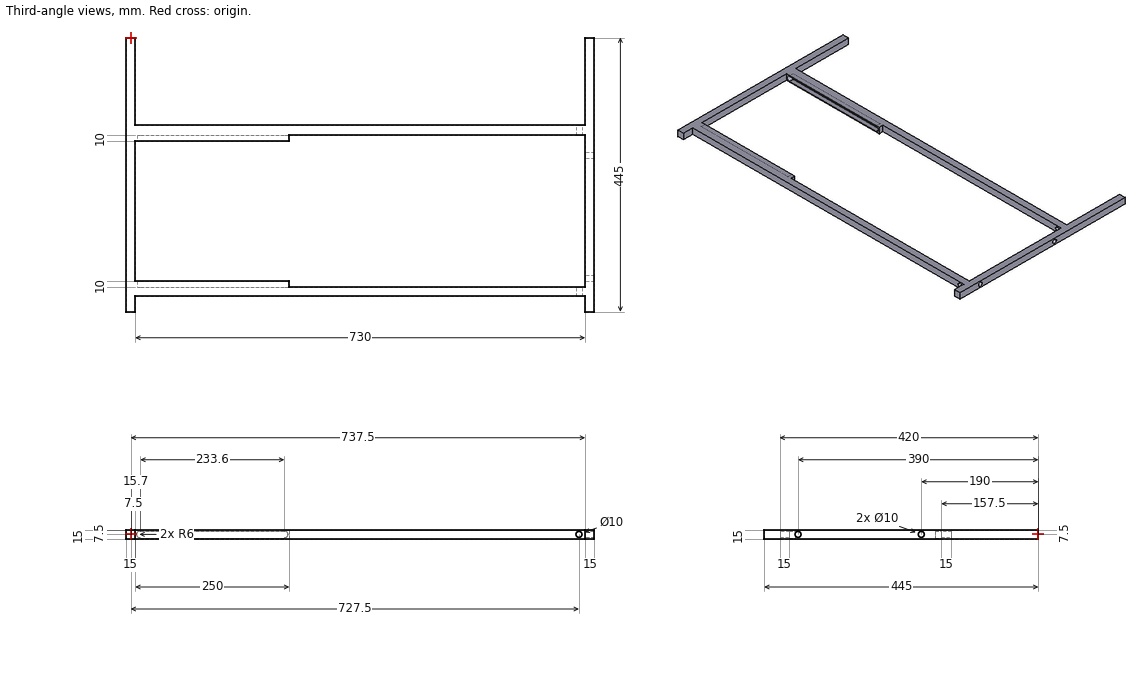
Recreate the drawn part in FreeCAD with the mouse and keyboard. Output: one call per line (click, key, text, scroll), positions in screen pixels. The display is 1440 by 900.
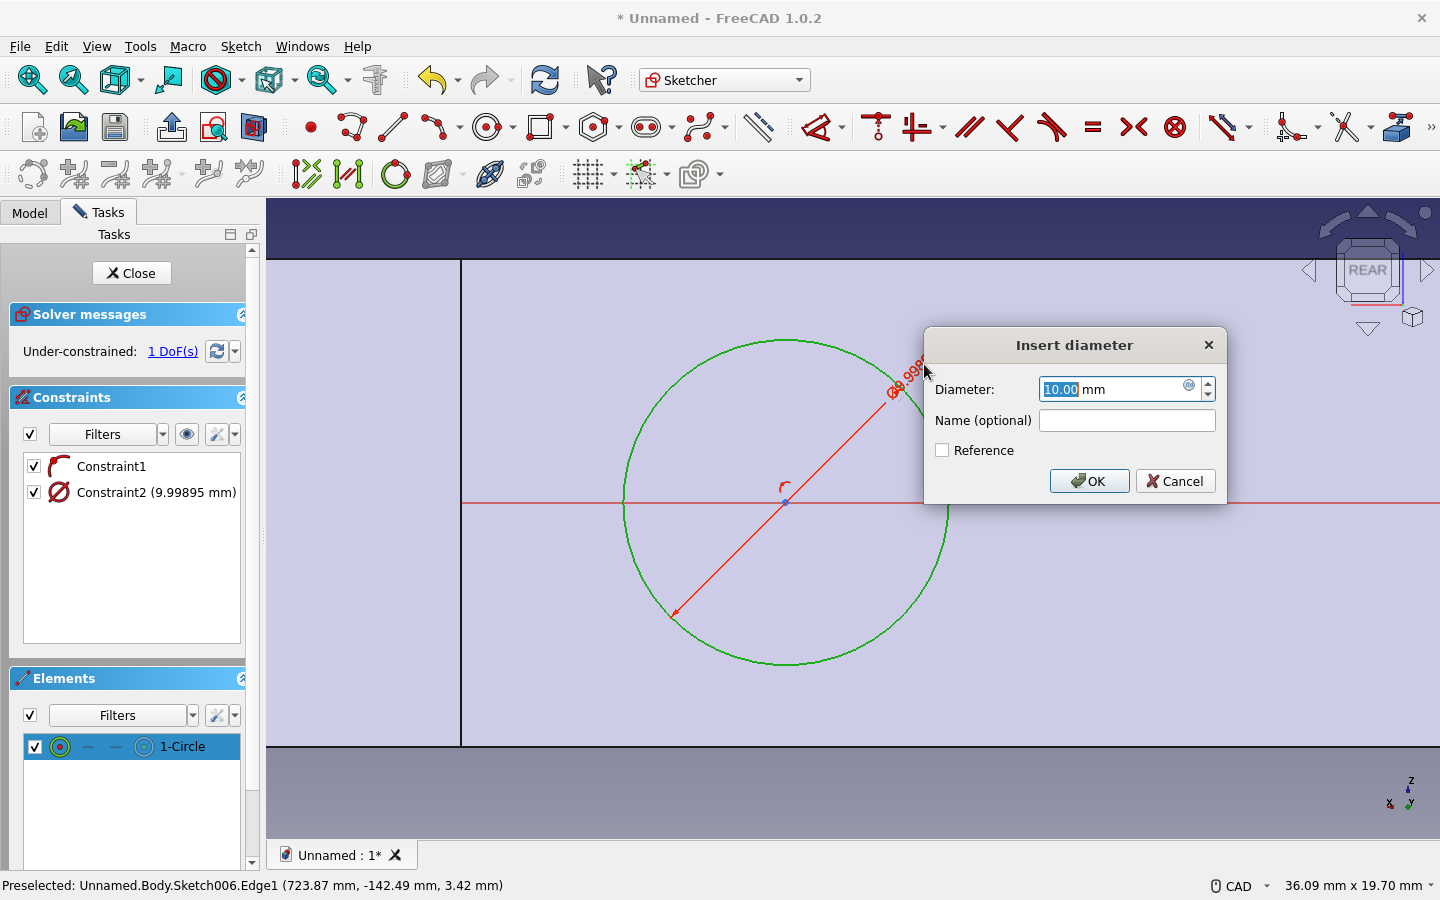
text(10)
key(Return)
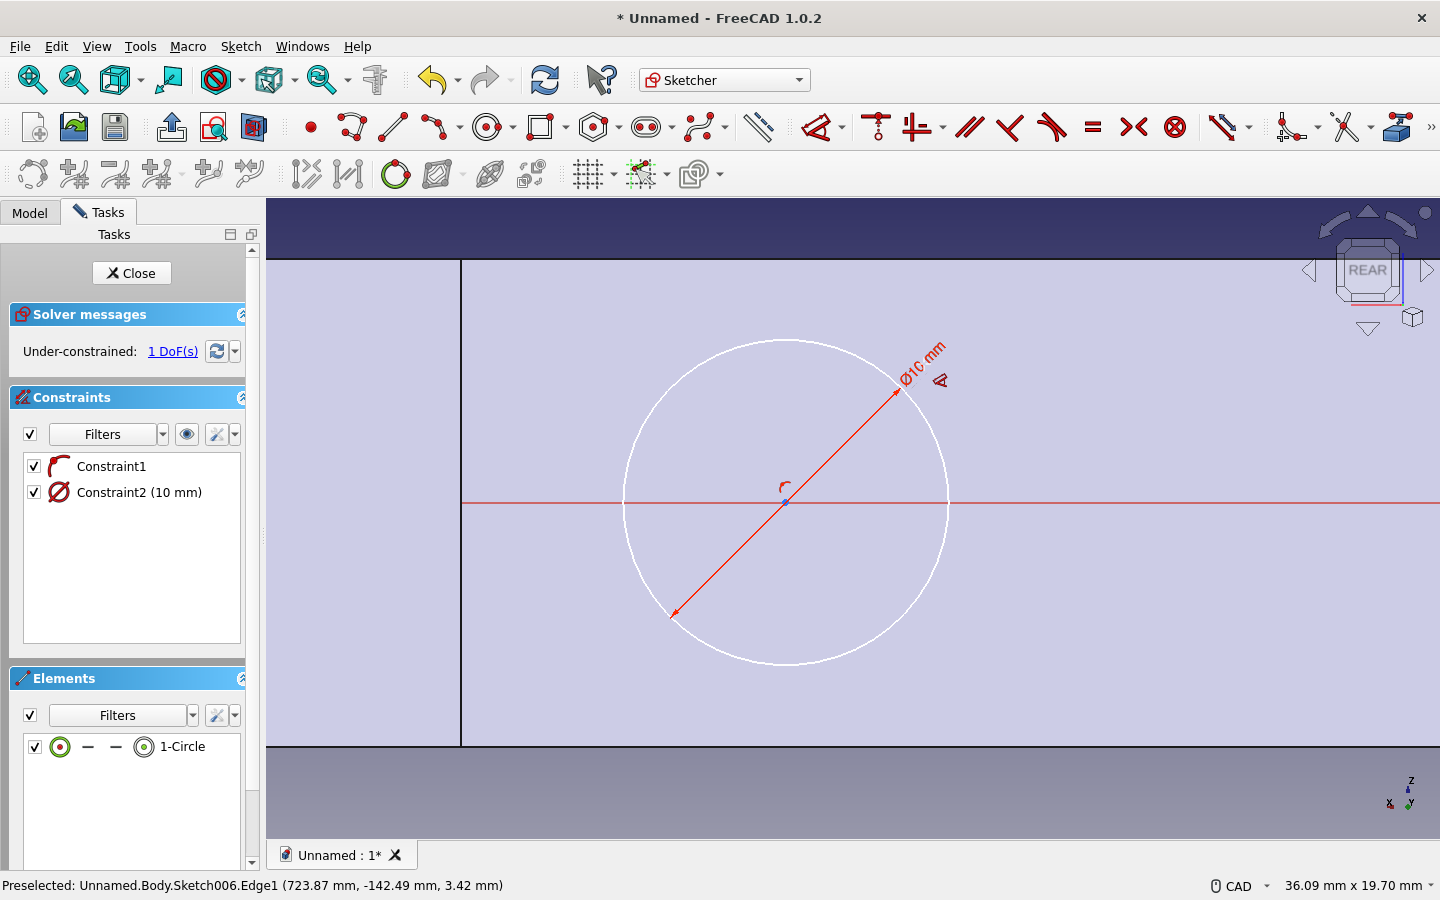
click(786, 503)
click(1030, 537)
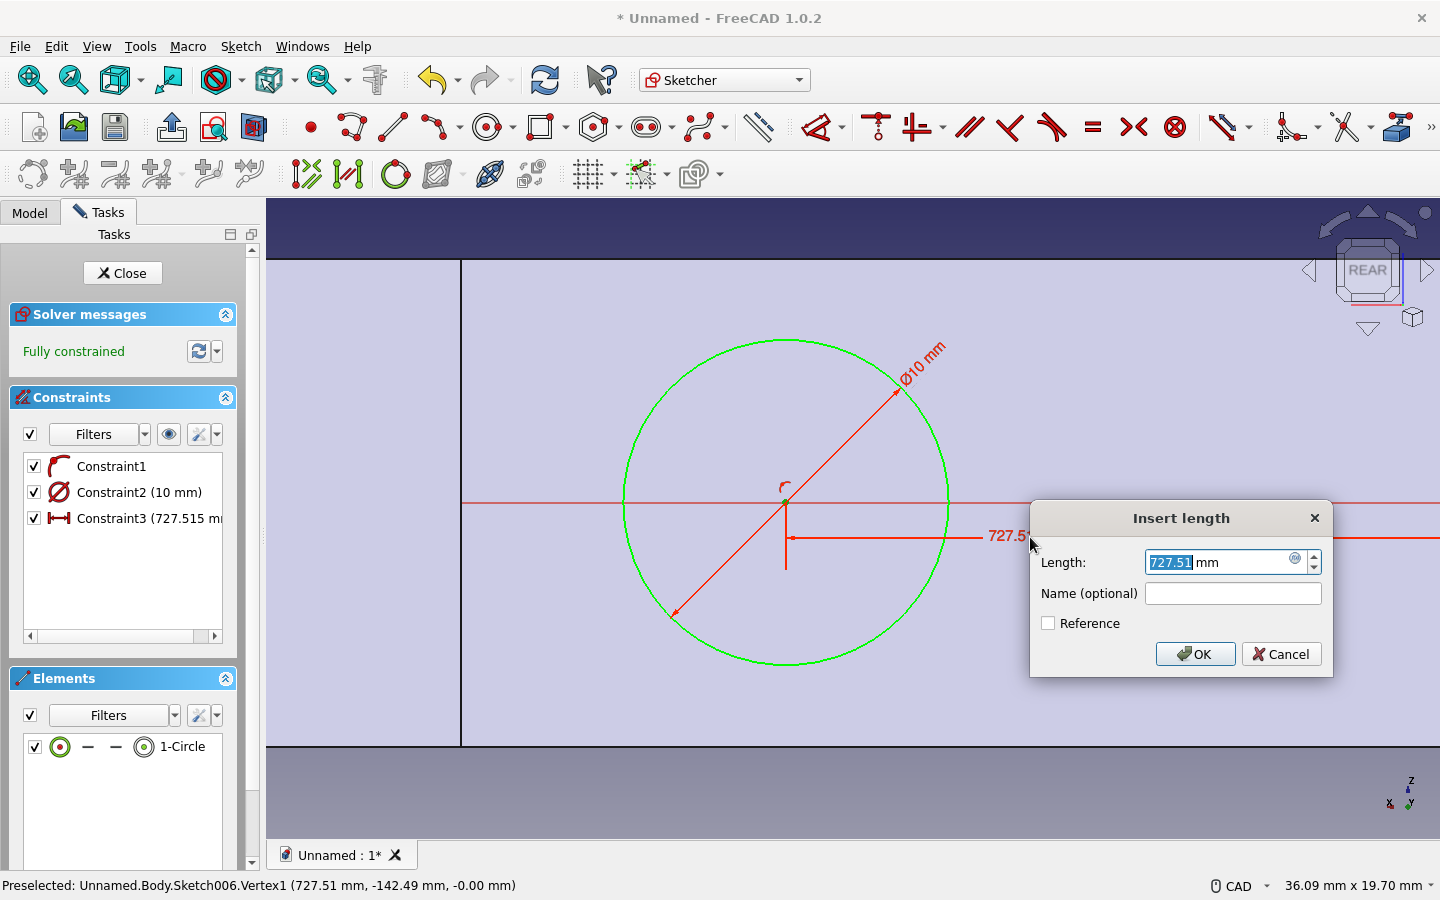
text(727.5)
key(Return)
key(Escape)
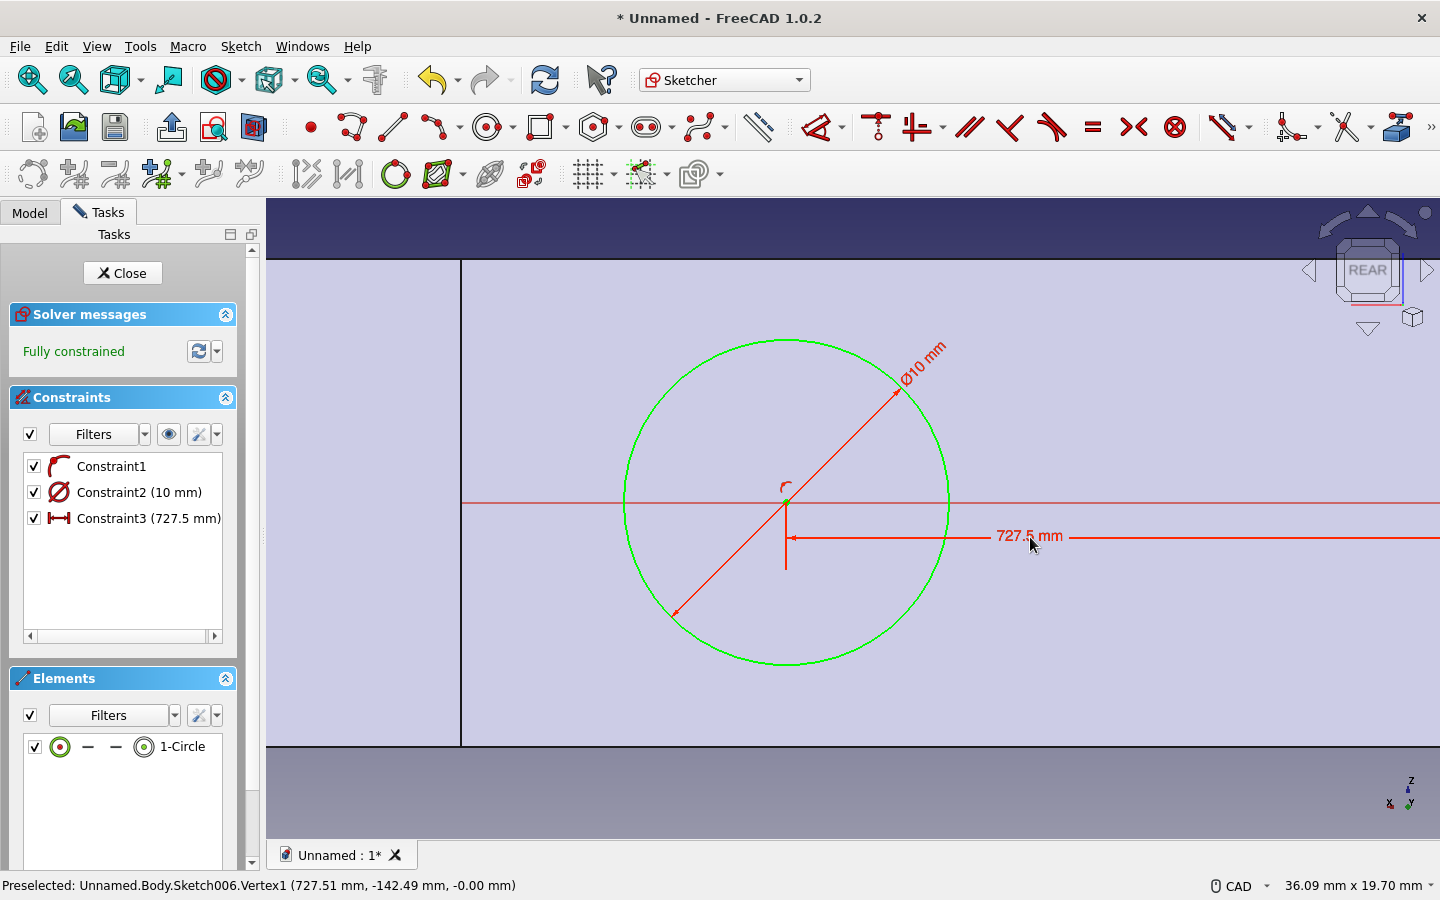
click(123, 273)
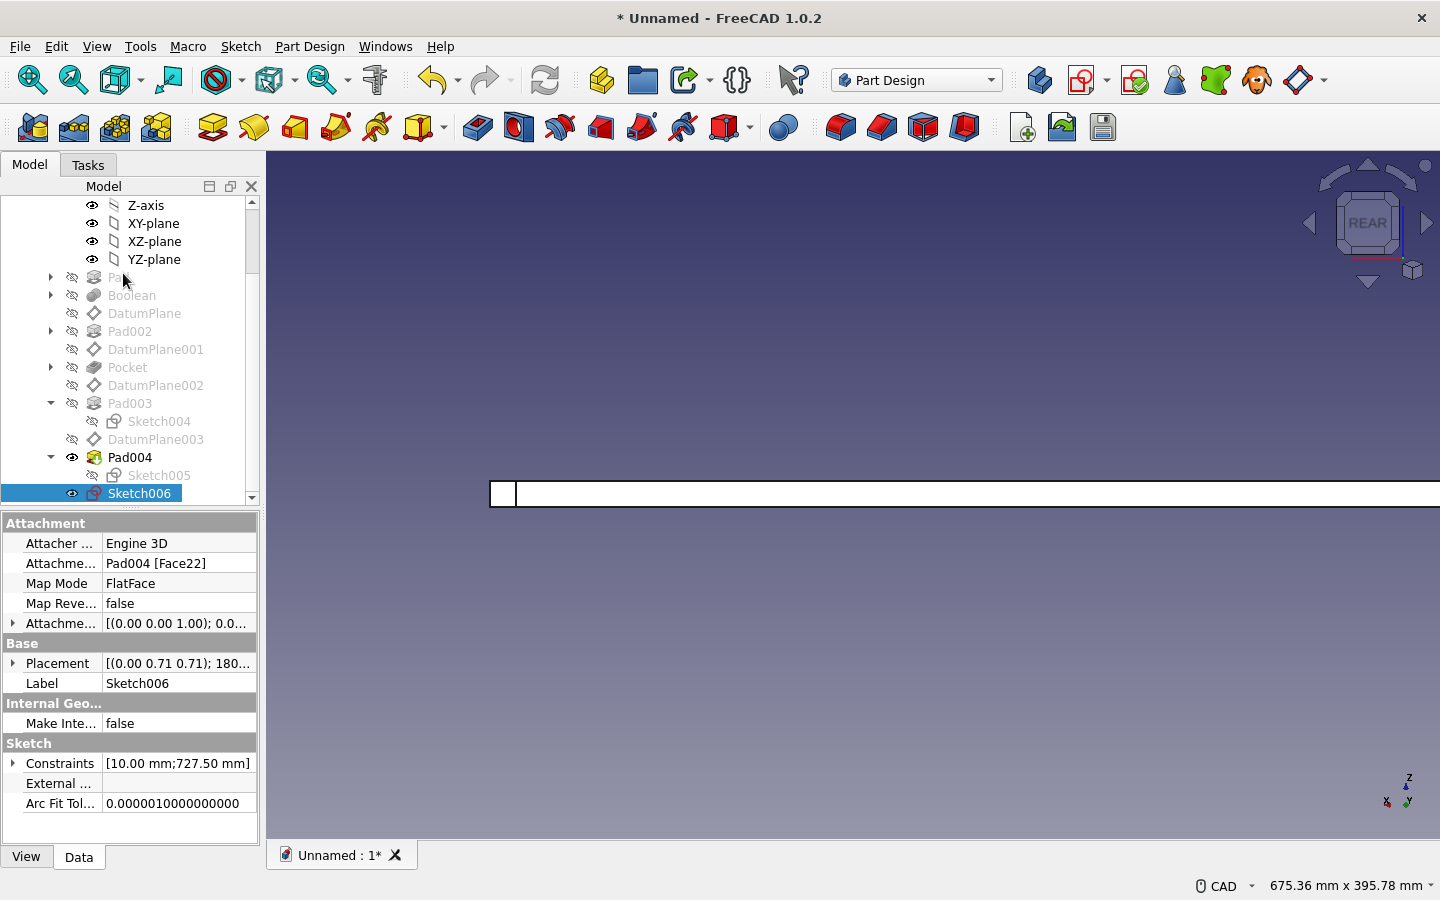
click(478, 128)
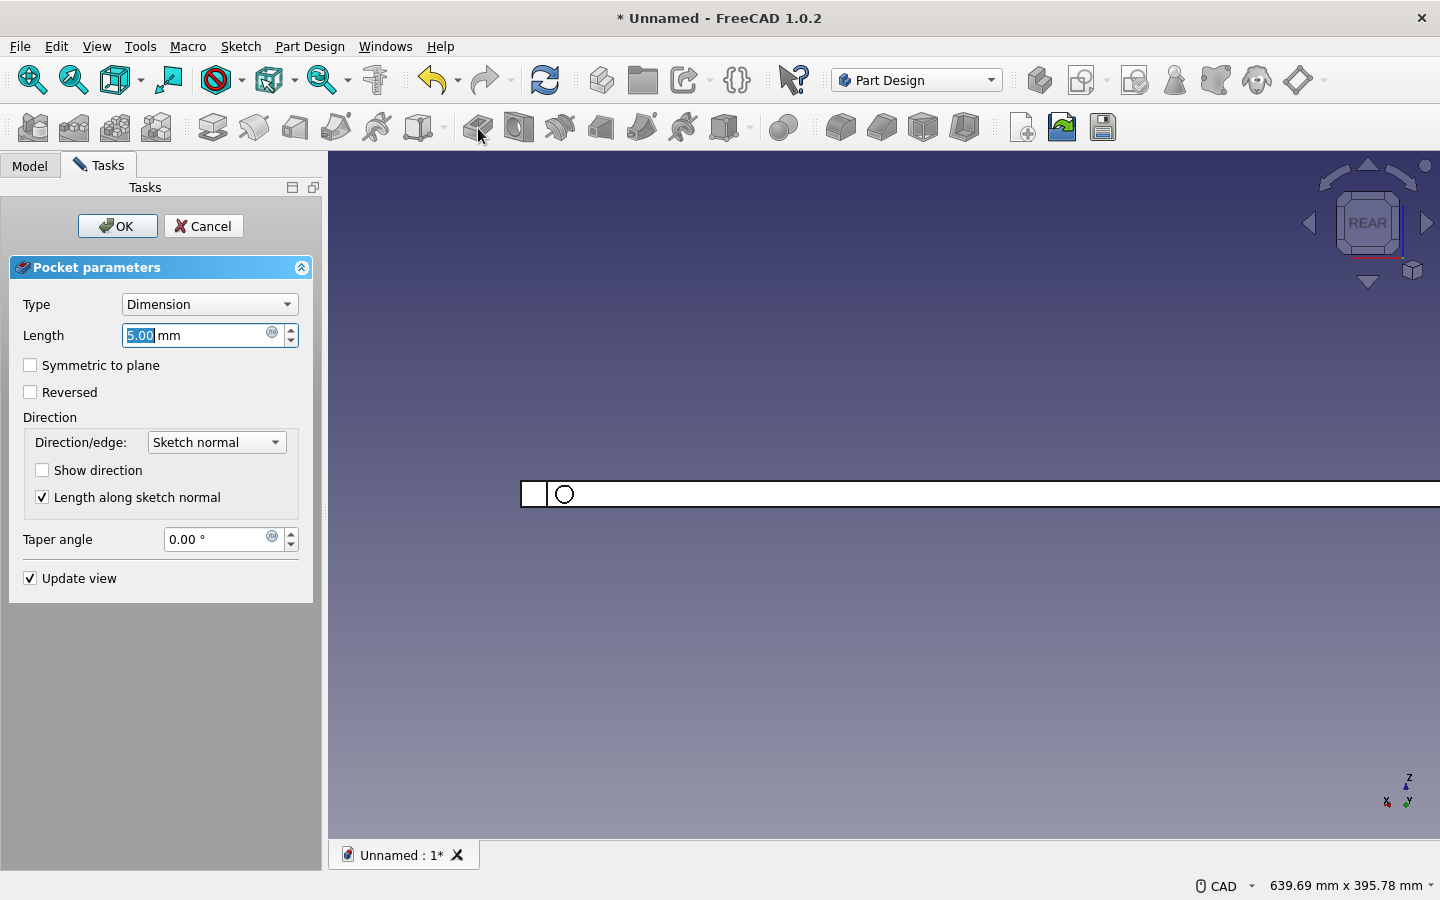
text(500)
key(Tab)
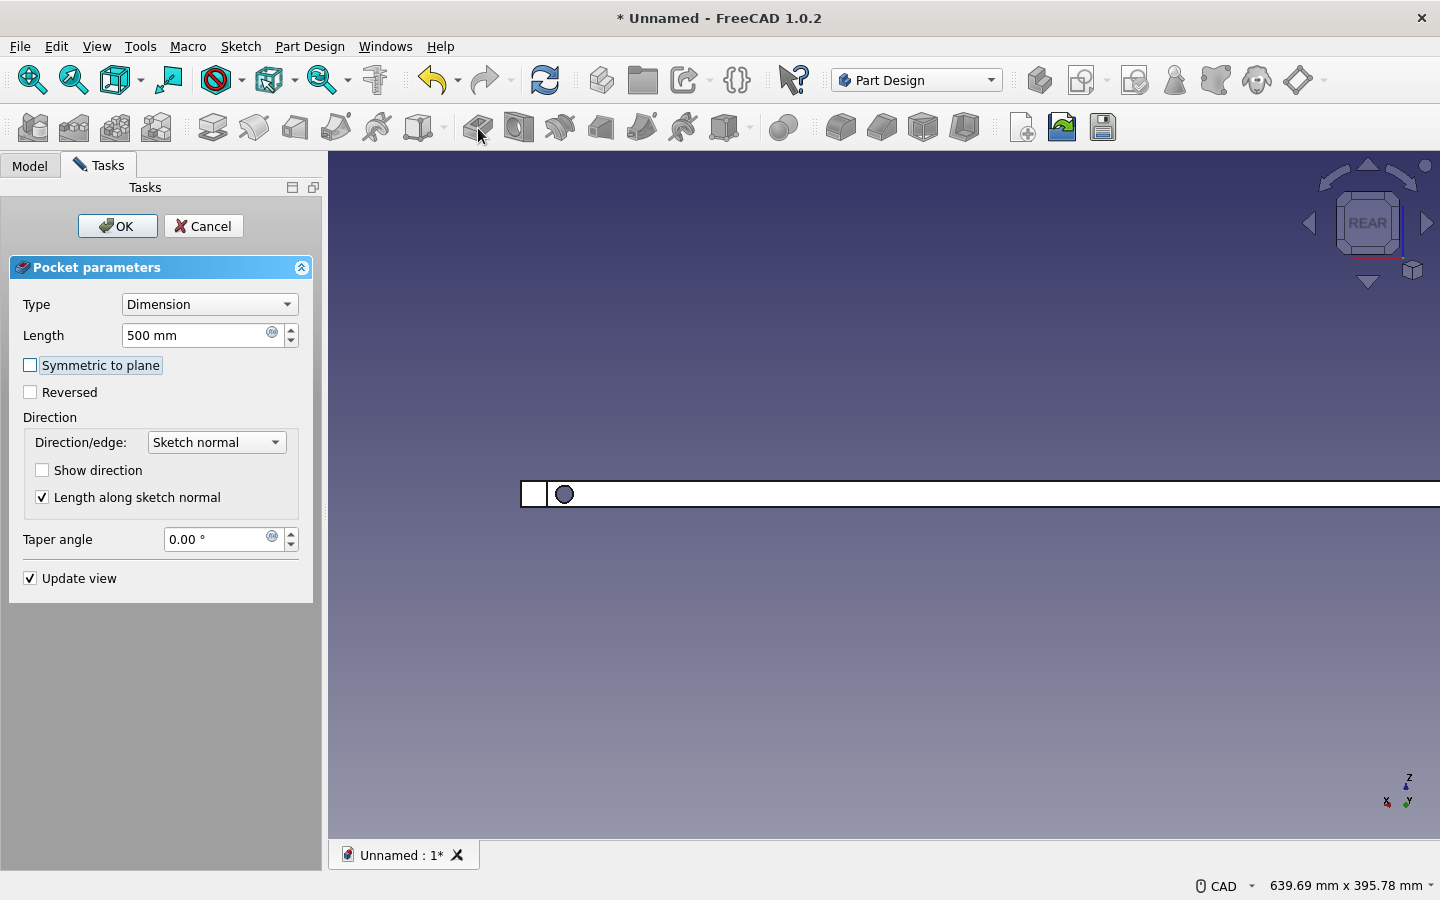
click(118, 226)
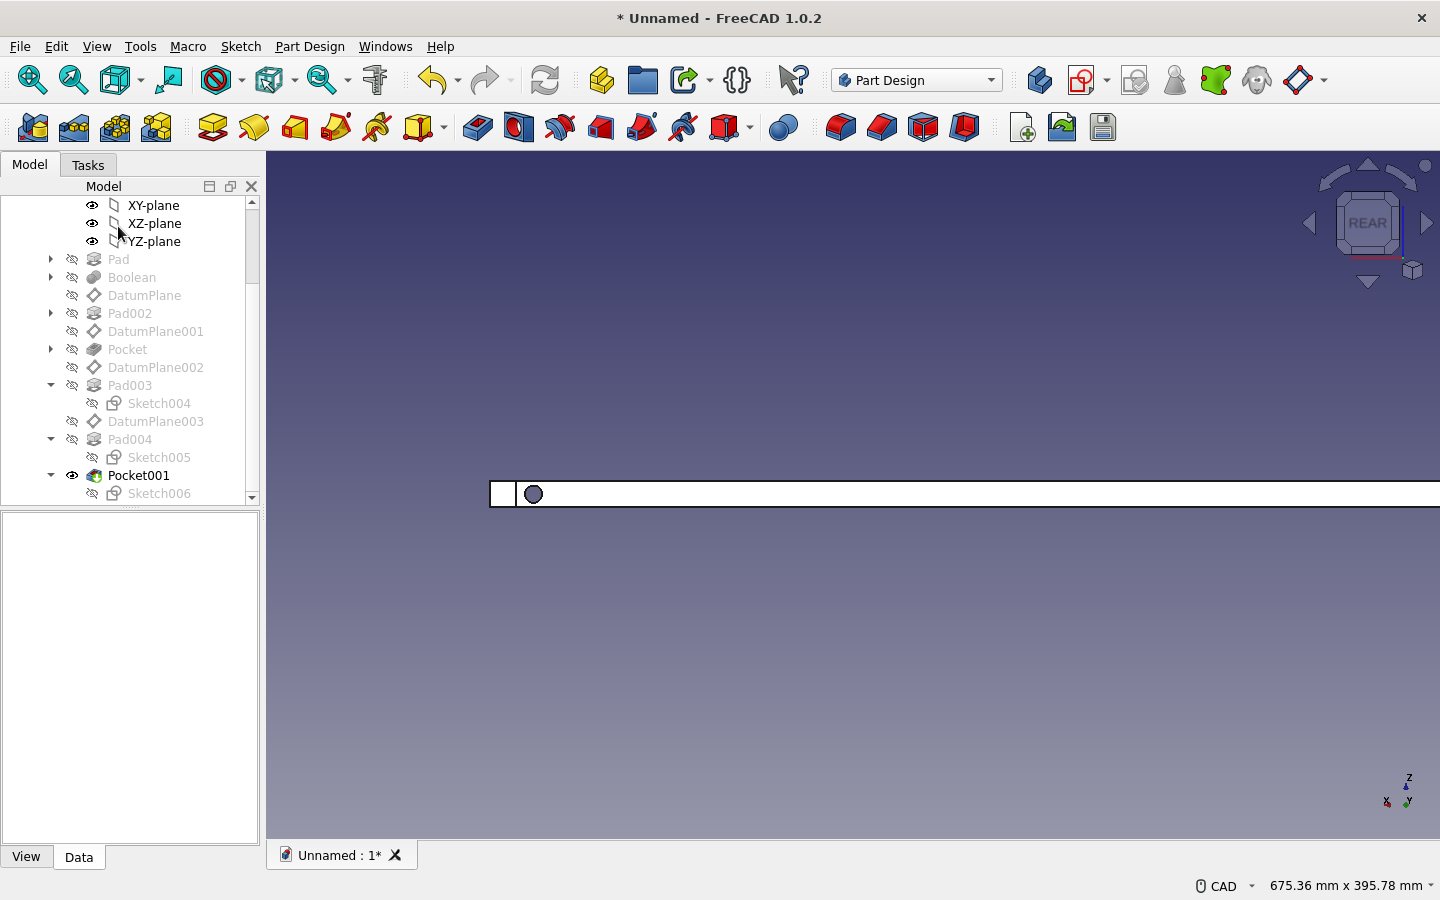
key(0)